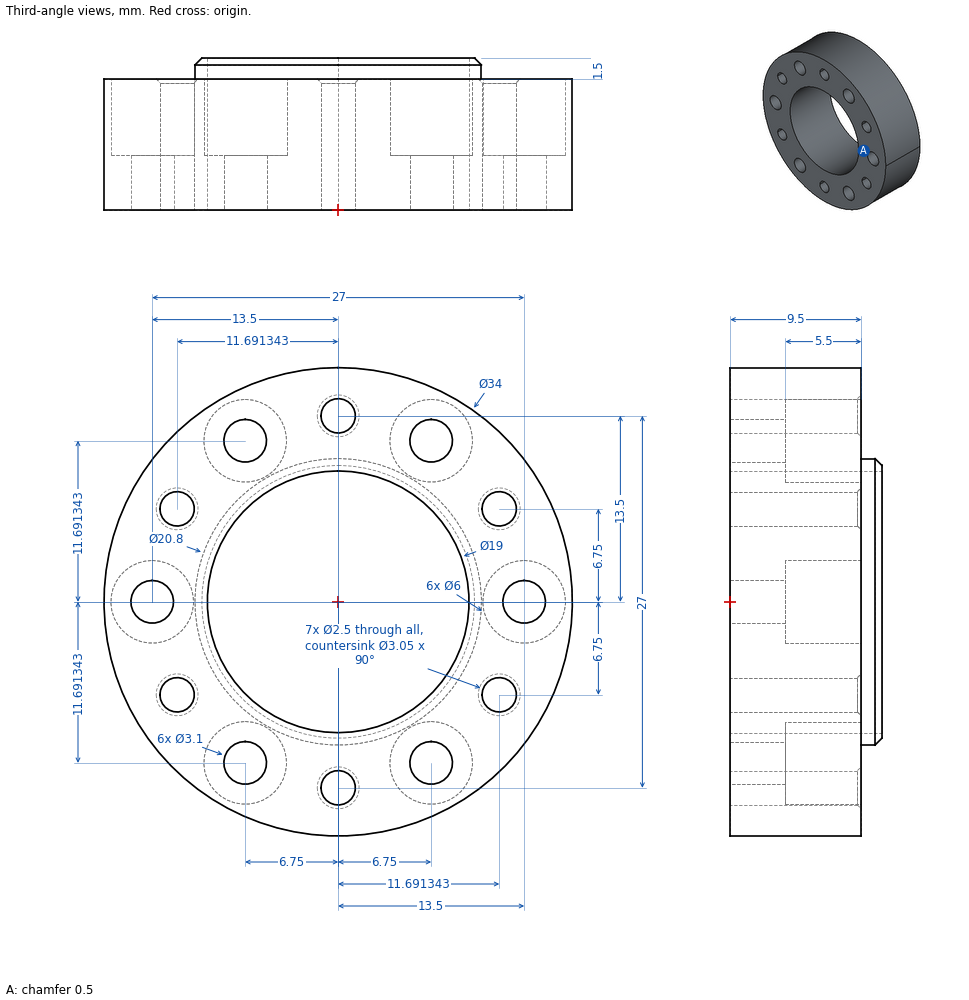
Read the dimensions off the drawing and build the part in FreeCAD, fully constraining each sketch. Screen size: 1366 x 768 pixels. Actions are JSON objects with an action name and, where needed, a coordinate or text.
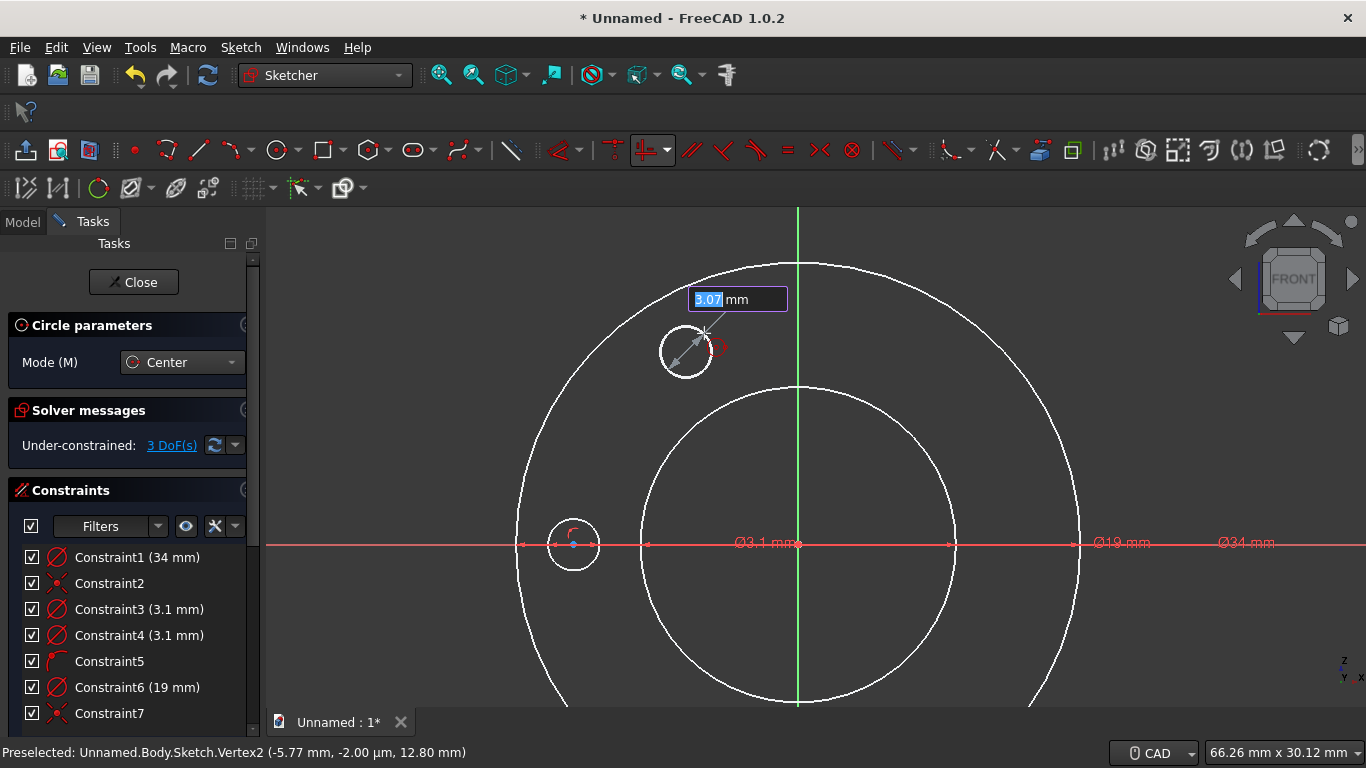
{"action": "type", "text": "3.1"}
{"action": "key", "text": "Return"}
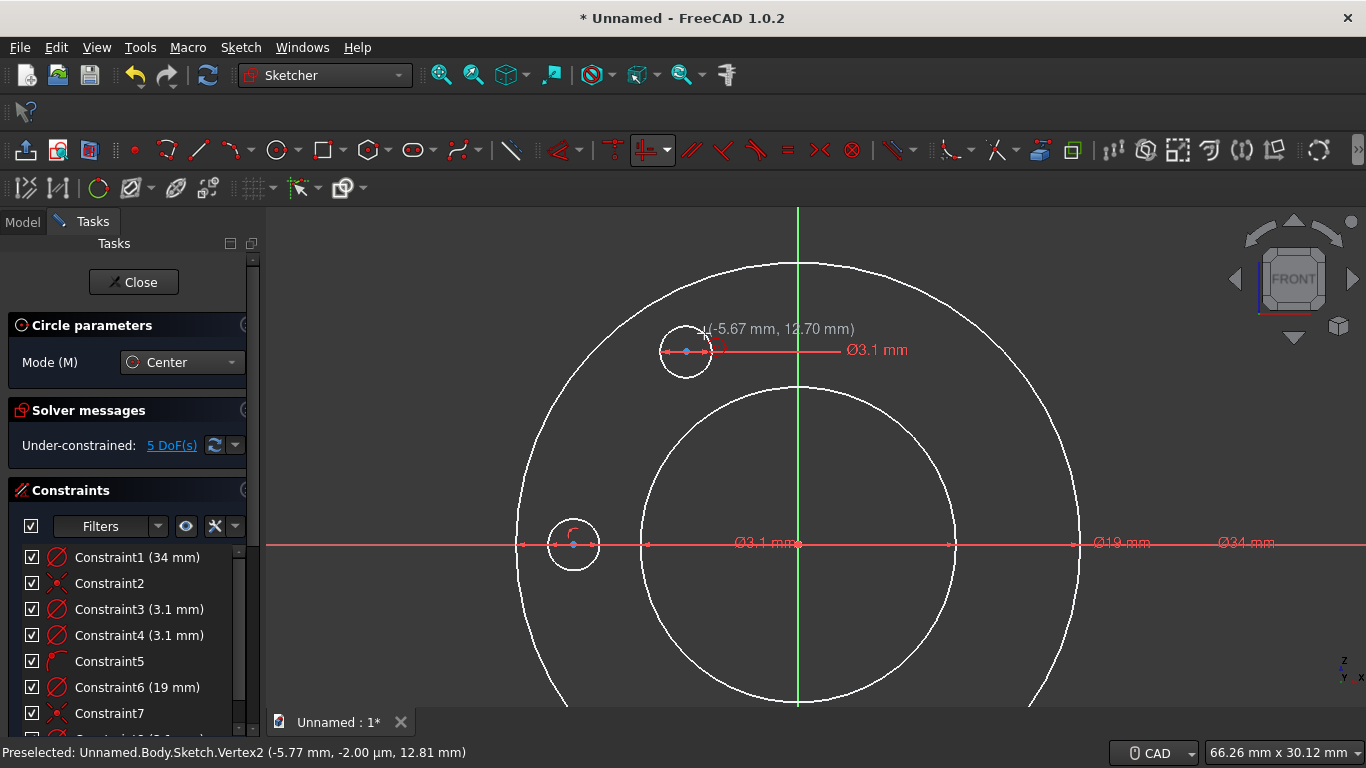
{"action": "scroll", "coordinate": [686, 350], "scroll_direction": "down", "scroll_amount": 3}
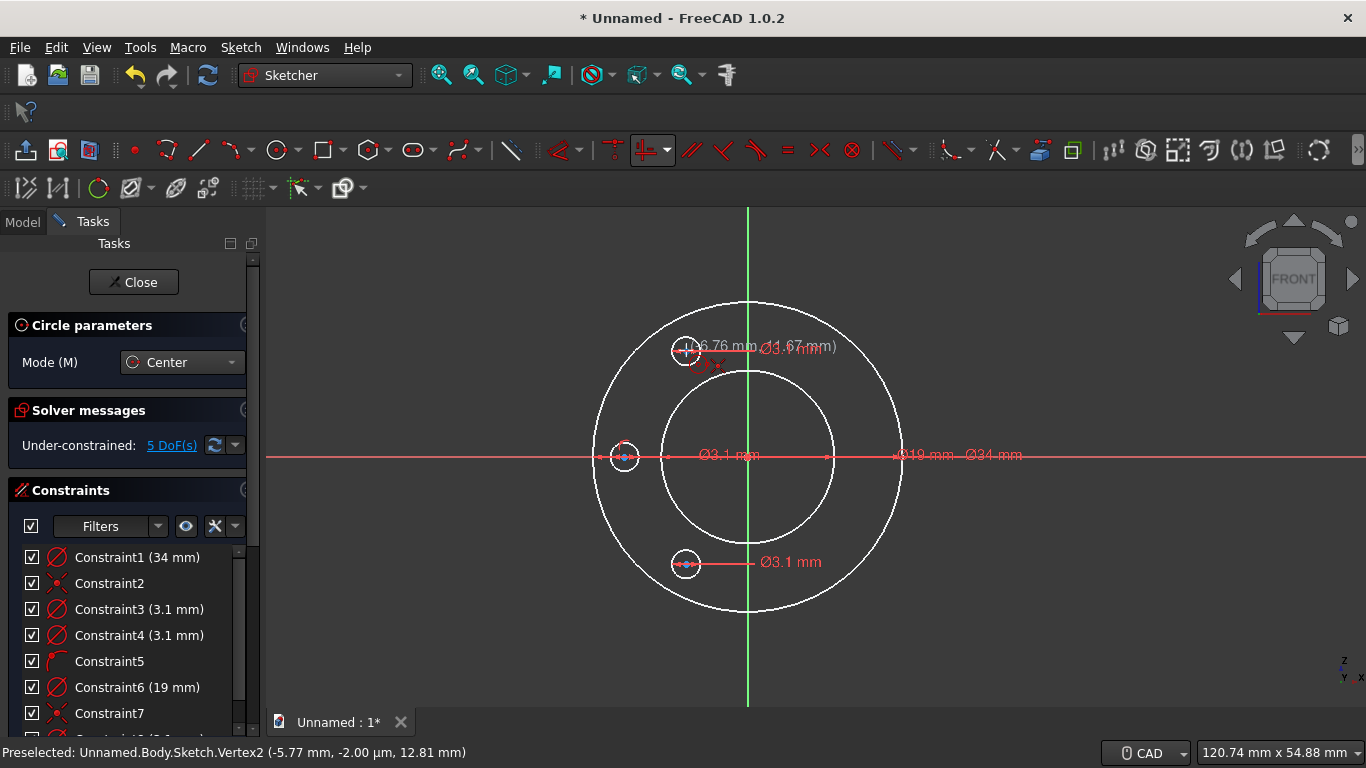
{"action": "scroll", "coordinate": [809, 564], "scroll_direction": "up", "scroll_amount": 3}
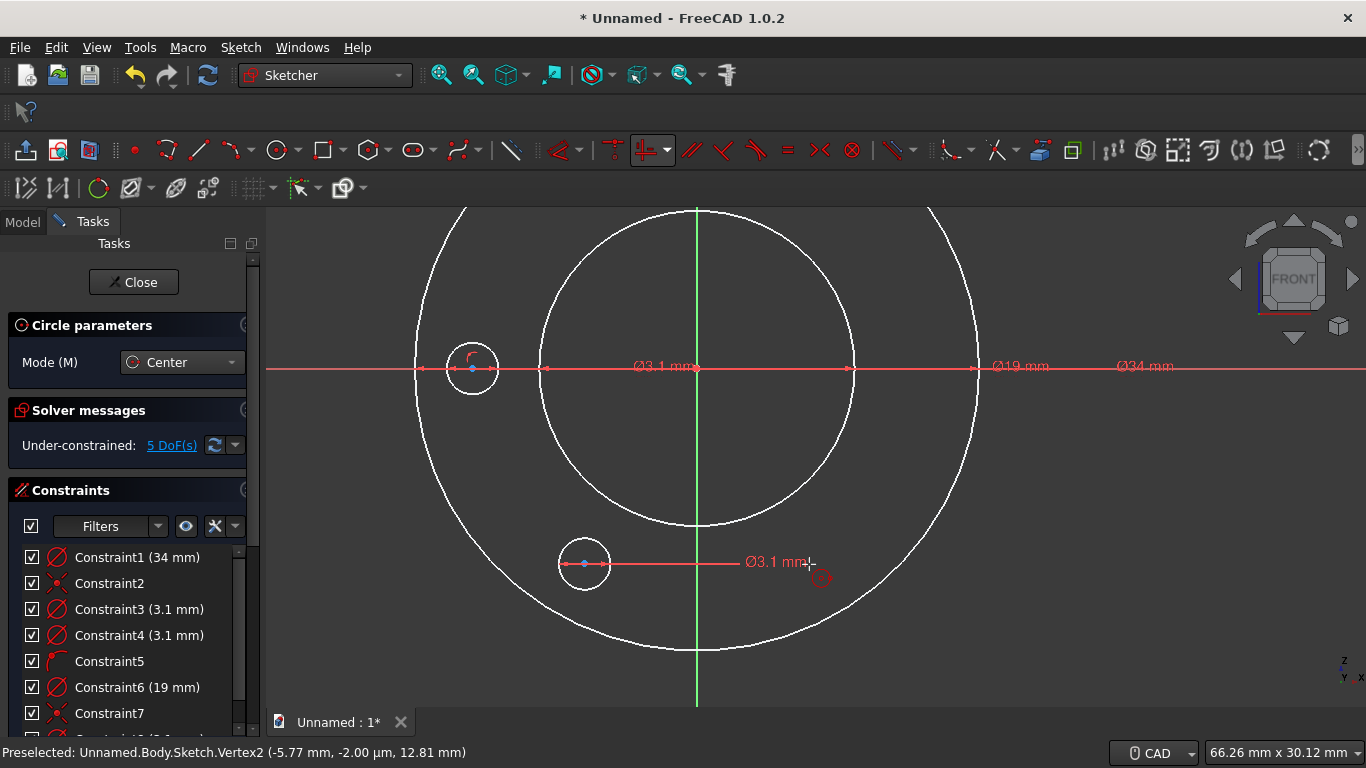
{"action": "left_click", "coordinate": [809, 563]}
{"action": "mouse_move", "coordinate": [827, 544]}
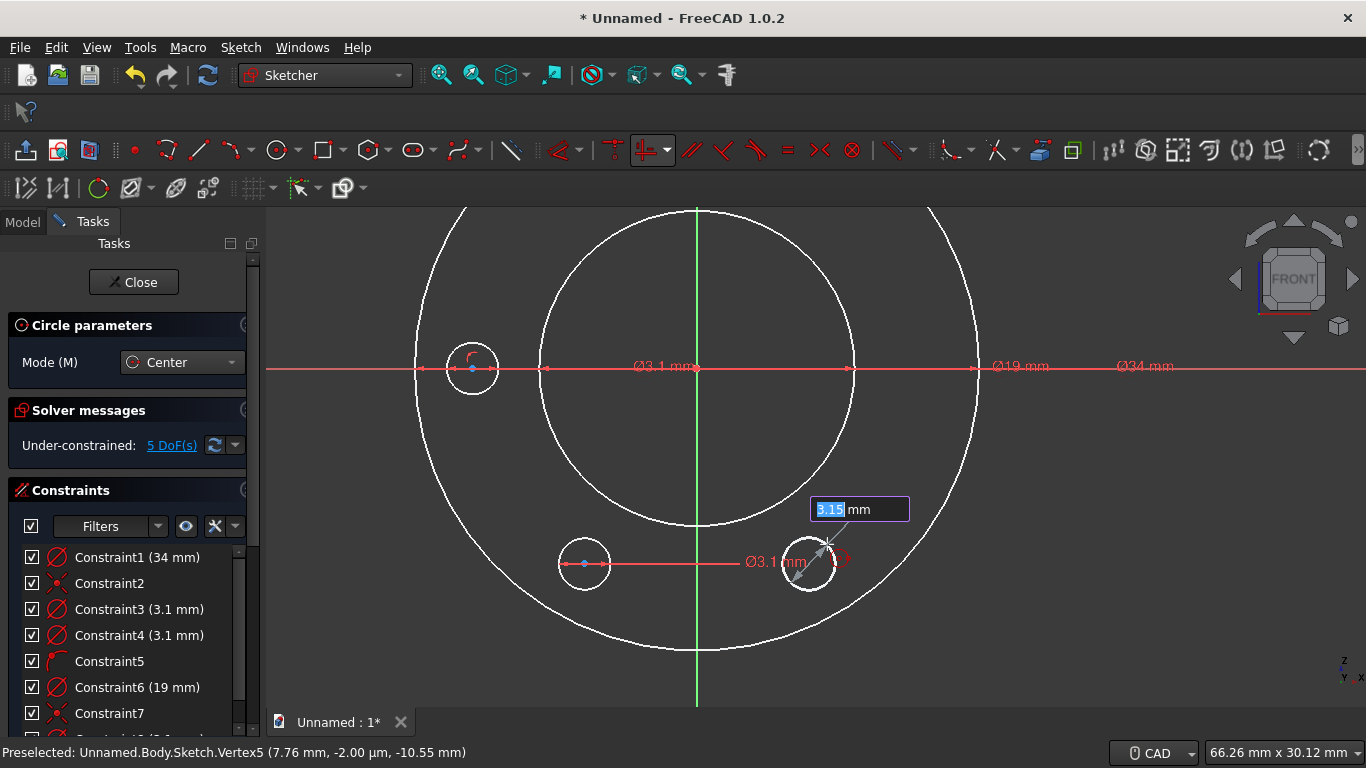
{"action": "type", "text": "3.1"}
{"action": "key", "text": "Return"}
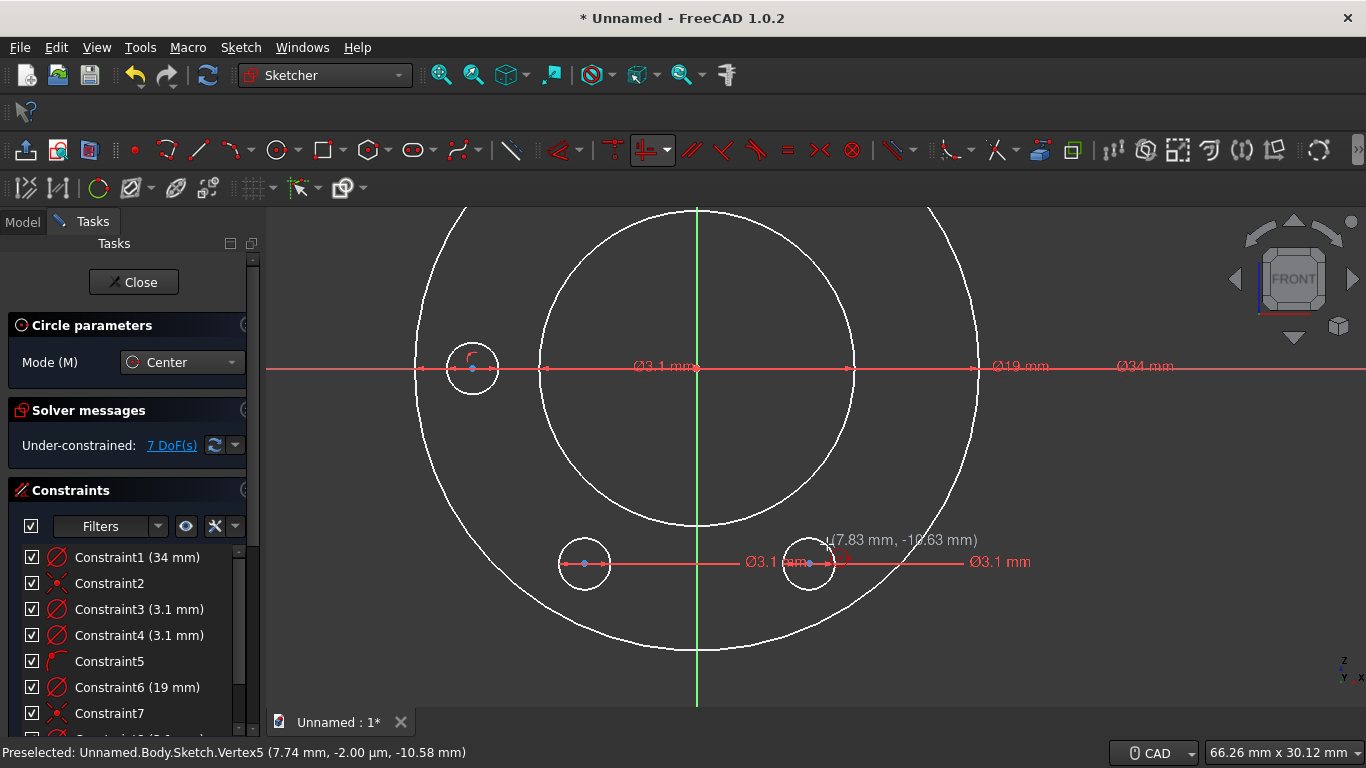
{"action": "left_click", "coordinate": [921, 369]}
{"action": "mouse_move", "coordinate": [939, 350]}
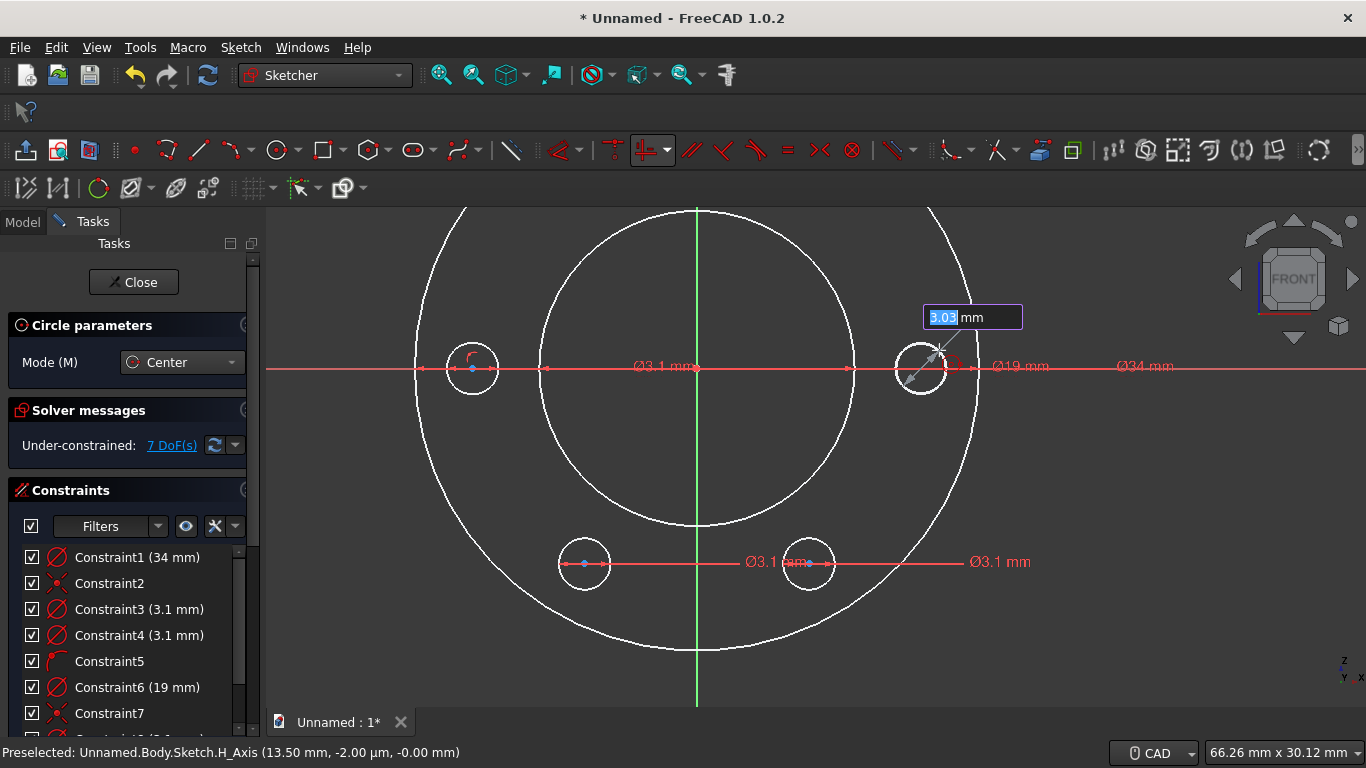
{"action": "type", "text": "3.1"}
{"action": "key", "text": "Return"}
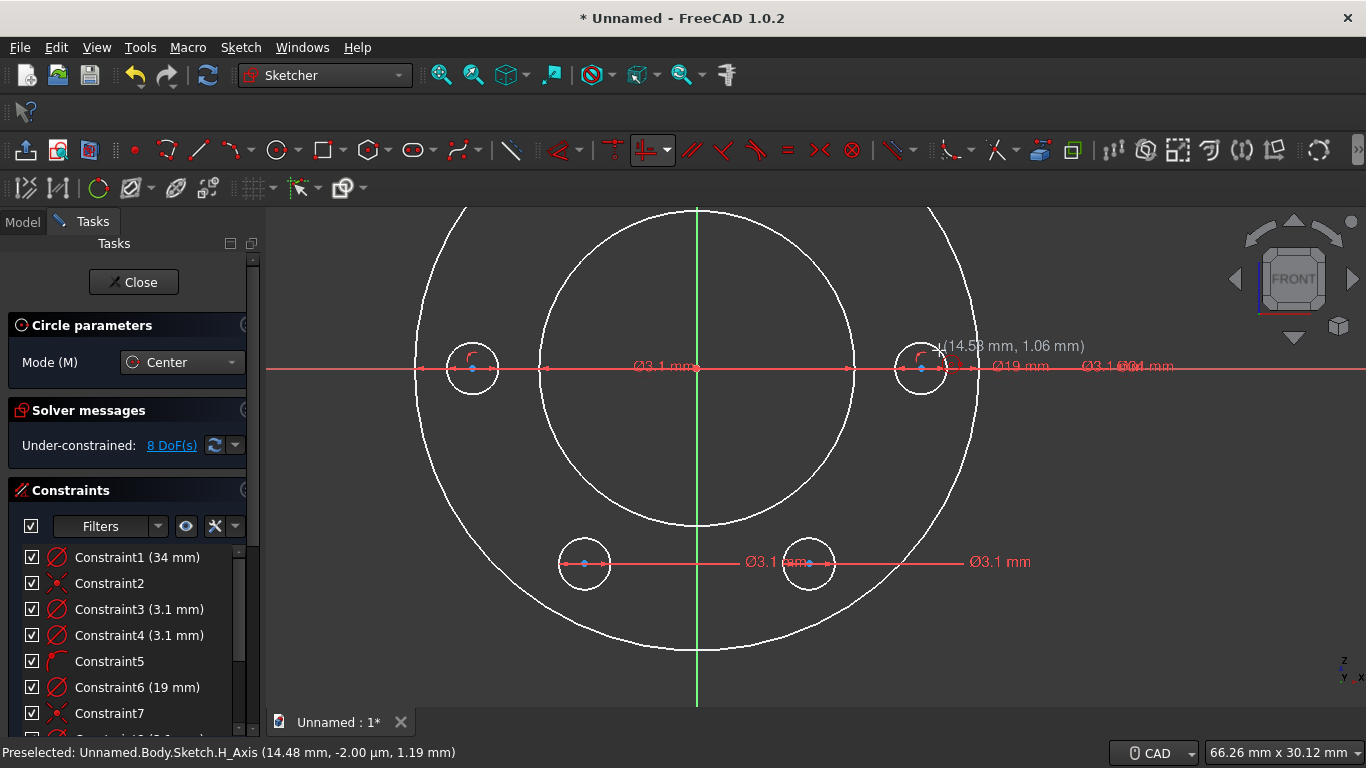
{"action": "scroll", "coordinate": [809, 565], "scroll_direction": "down", "scroll_amount": 3}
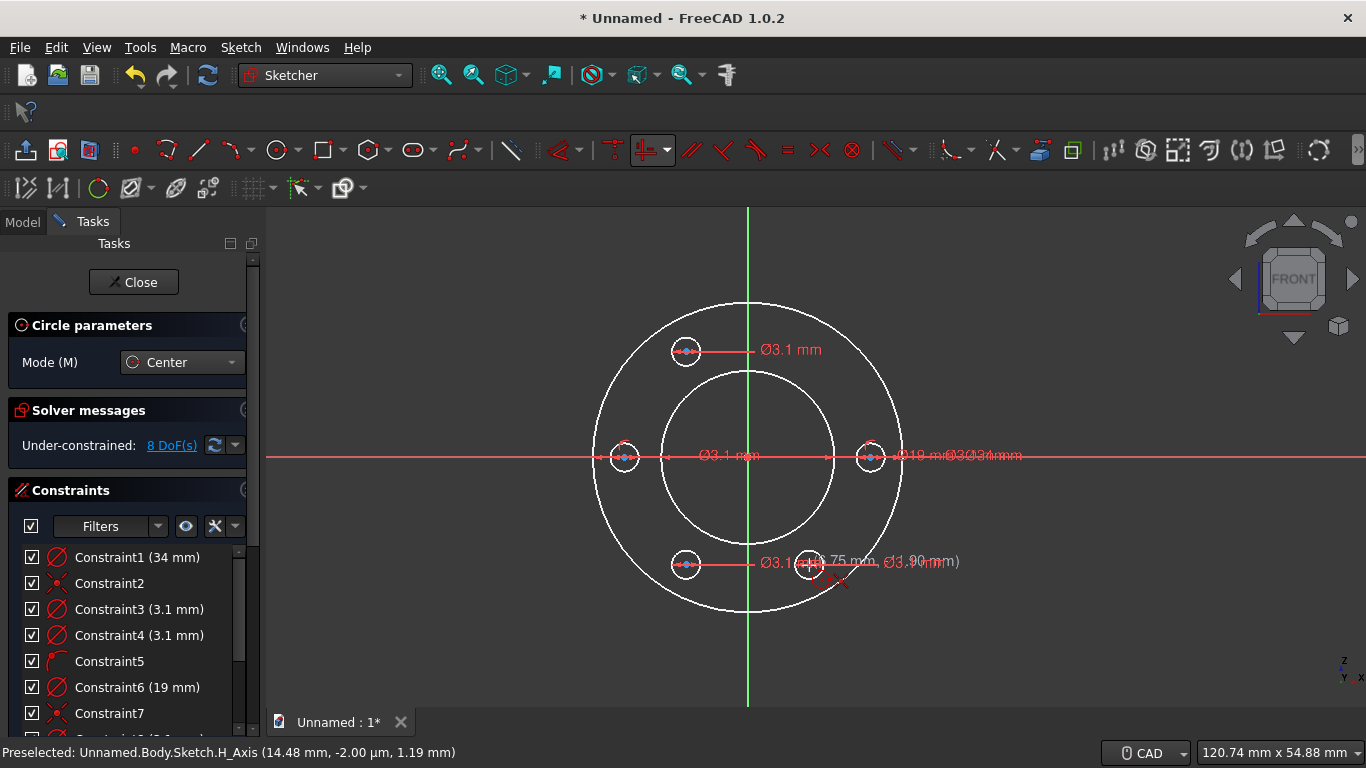
{"action": "scroll", "coordinate": [809, 351], "scroll_direction": "up", "scroll_amount": 3}